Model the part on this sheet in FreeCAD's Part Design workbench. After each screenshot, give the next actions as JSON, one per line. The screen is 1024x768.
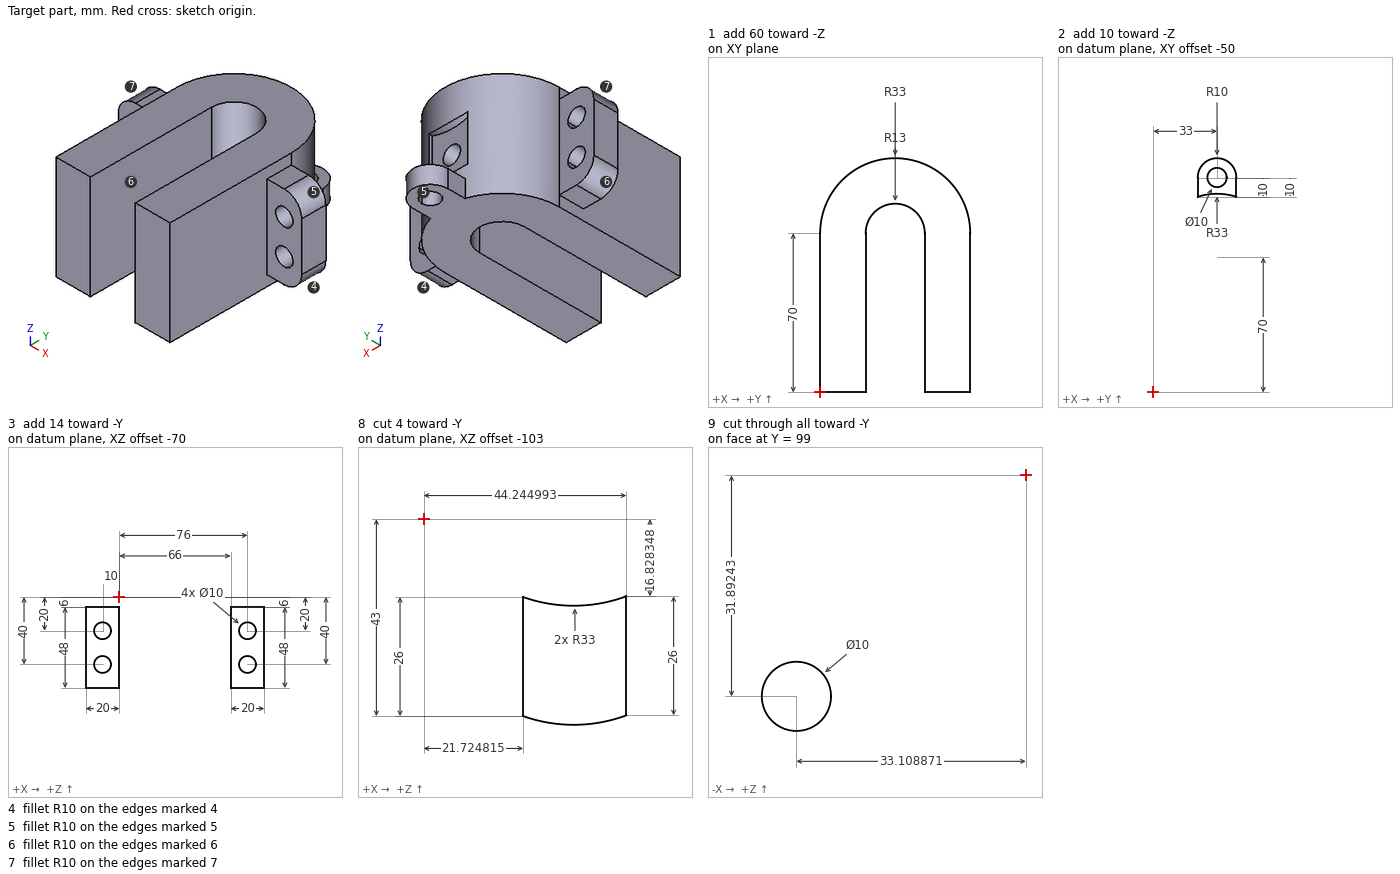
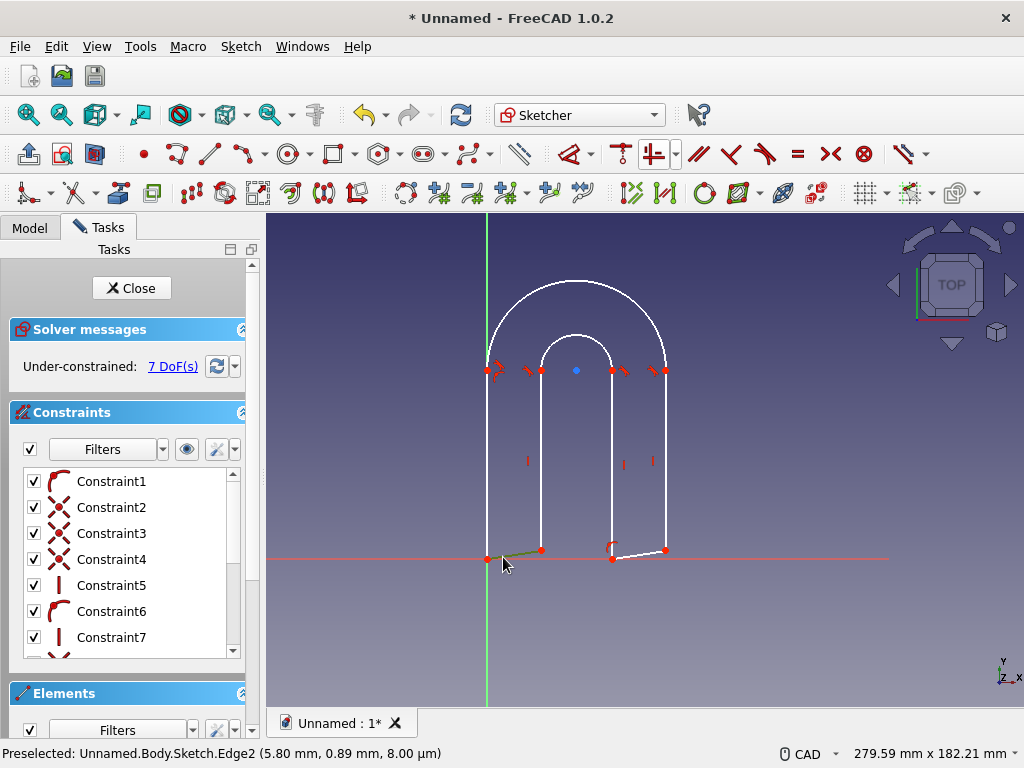
{"action": "key", "text": "h"}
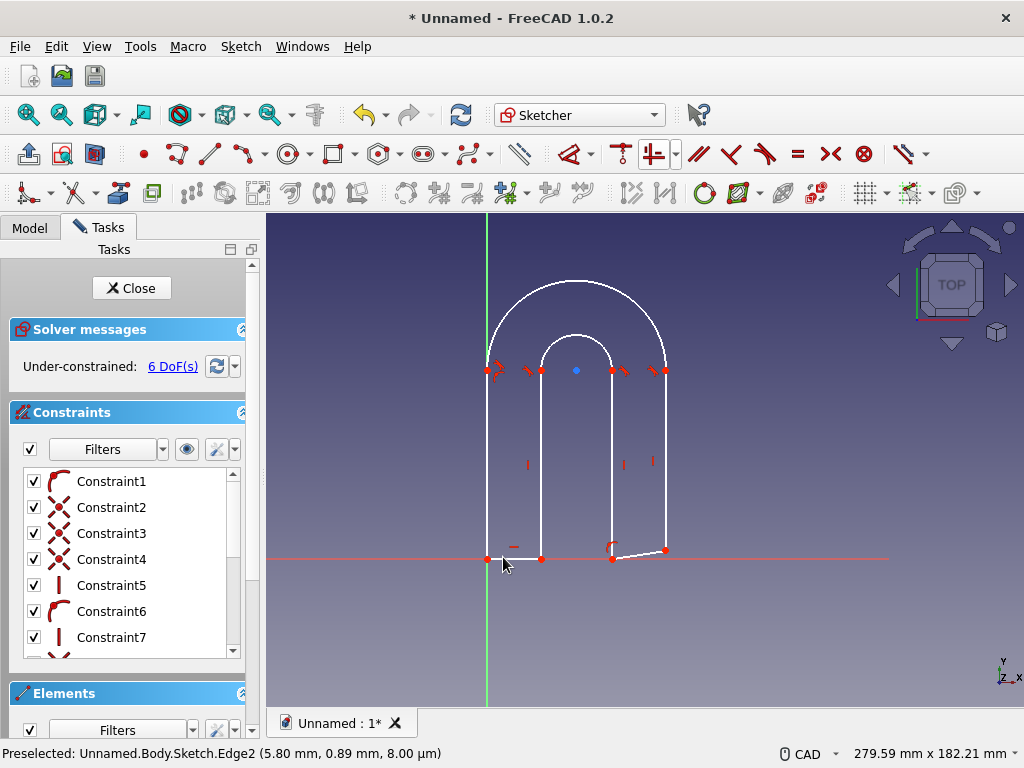
{"action": "left_click", "coordinate": [628, 557]}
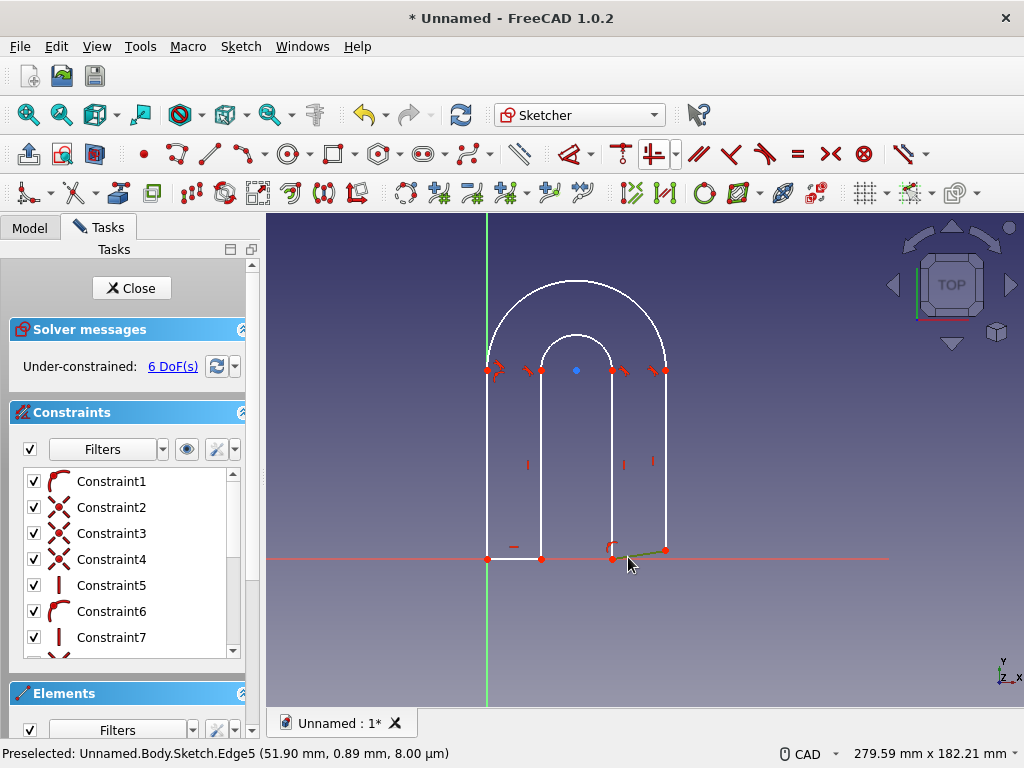
{"action": "key", "text": "h"}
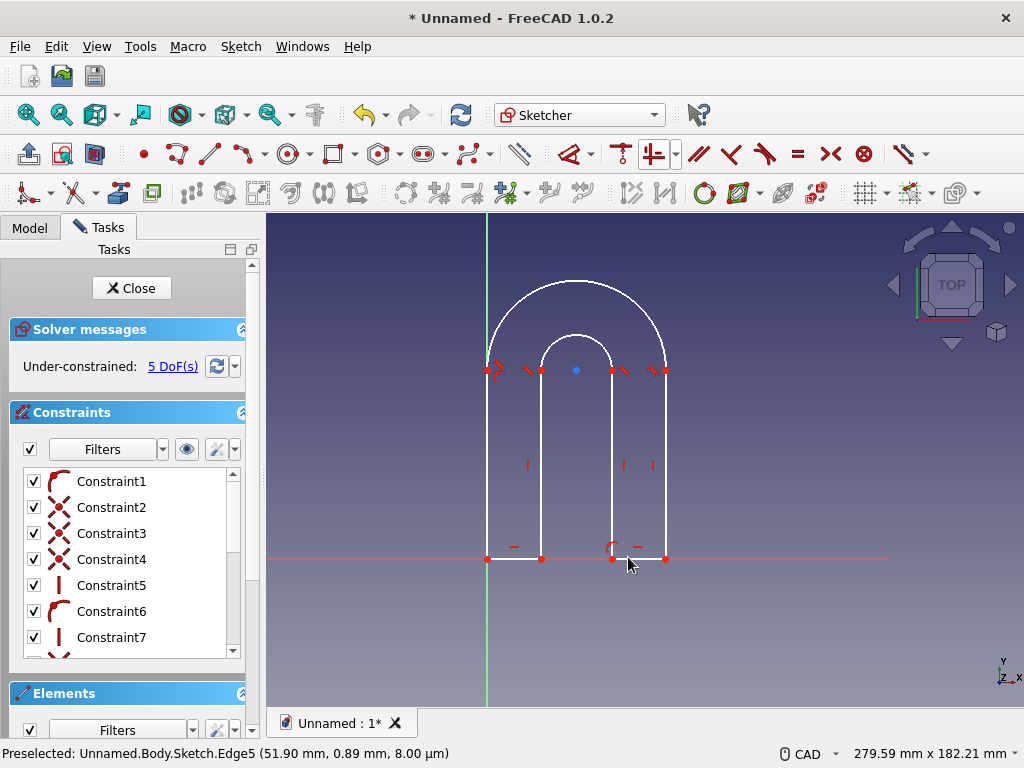
{"action": "left_click", "coordinate": [597, 342]}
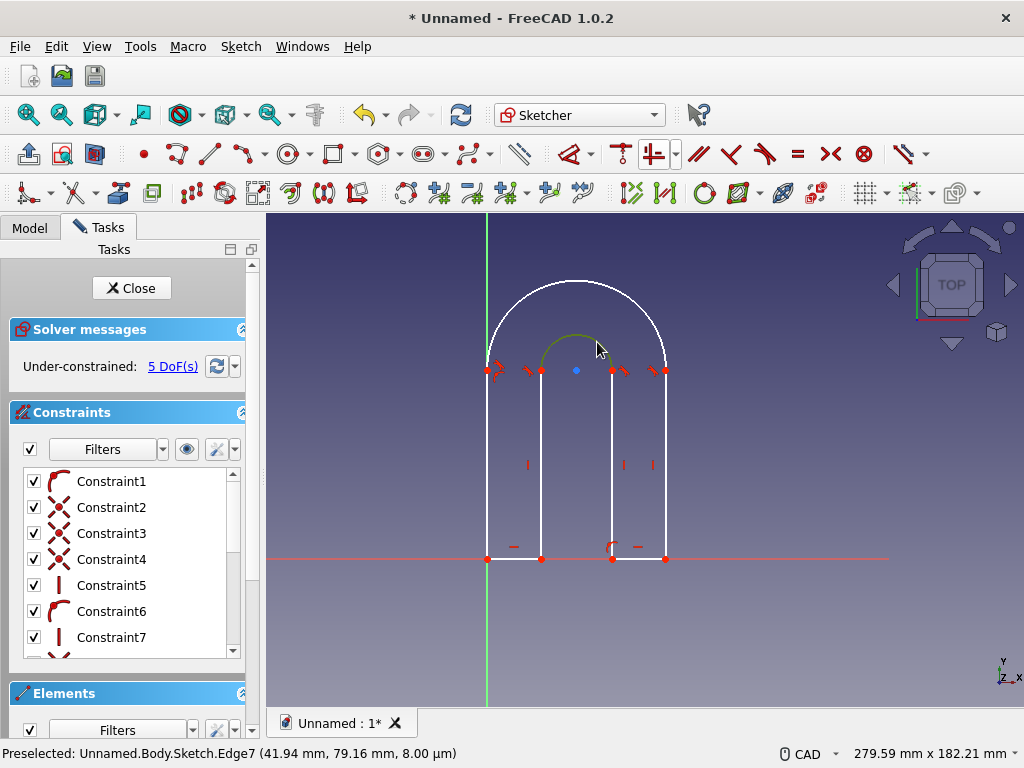
{"action": "left_click", "coordinate": [629, 298]}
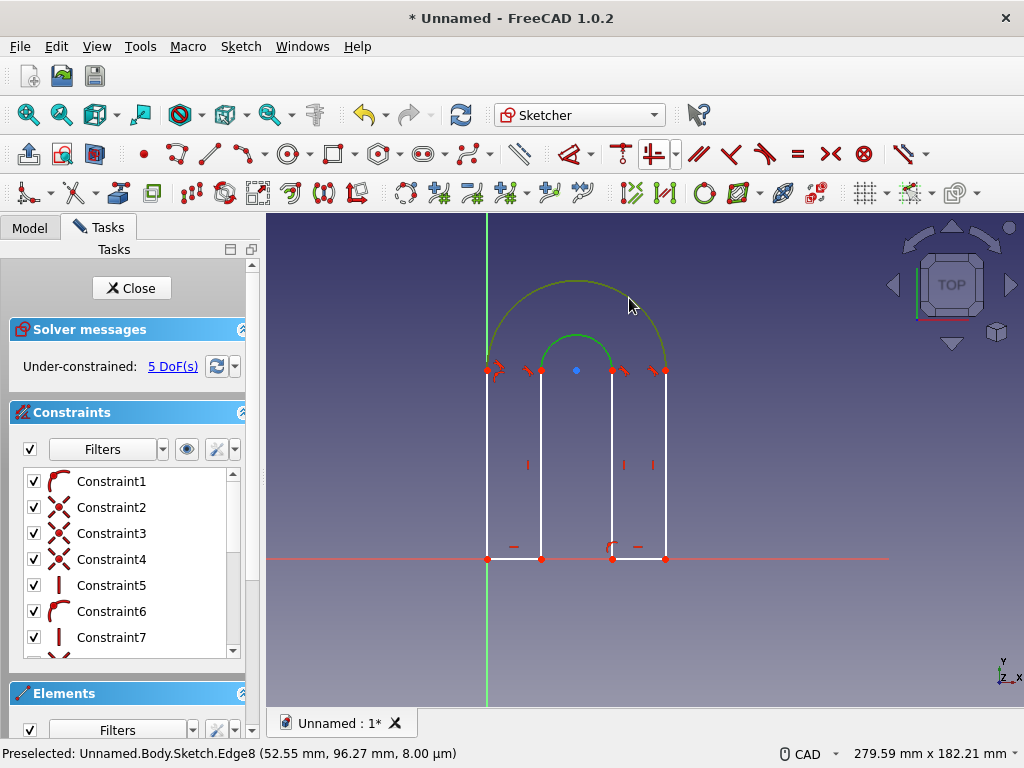
{"action": "left_click", "coordinate": [621, 154]}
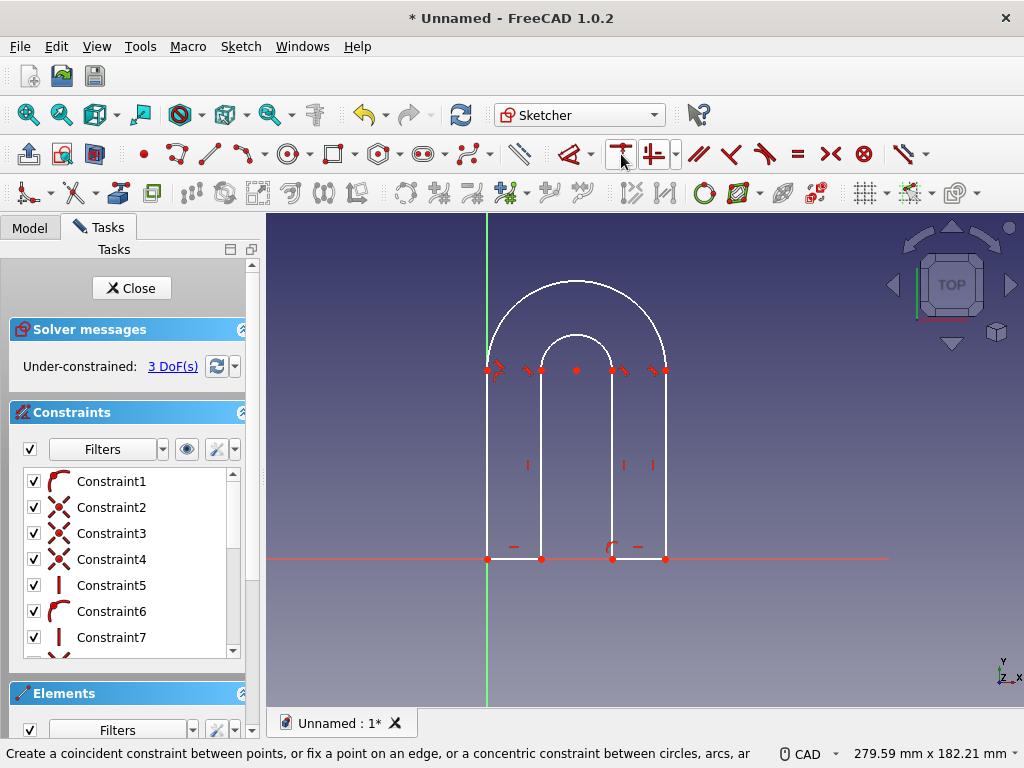
{"action": "left_click", "coordinate": [568, 154]}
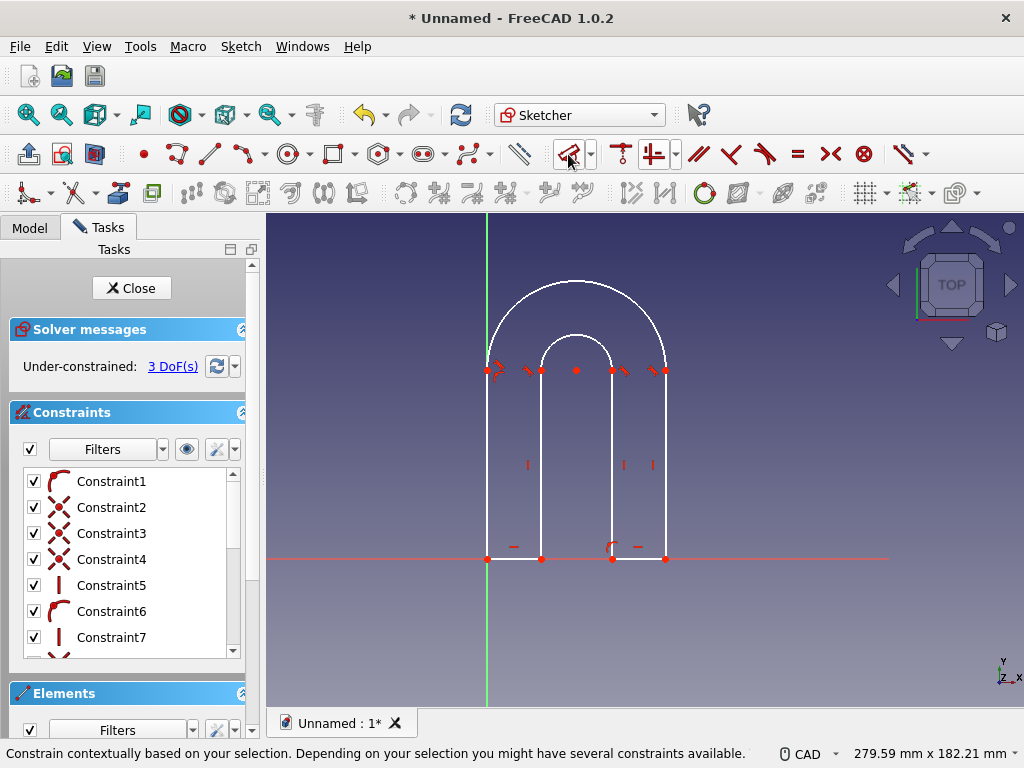
{"action": "left_click", "coordinate": [597, 342]}
{"action": "left_click", "coordinate": [616, 316]}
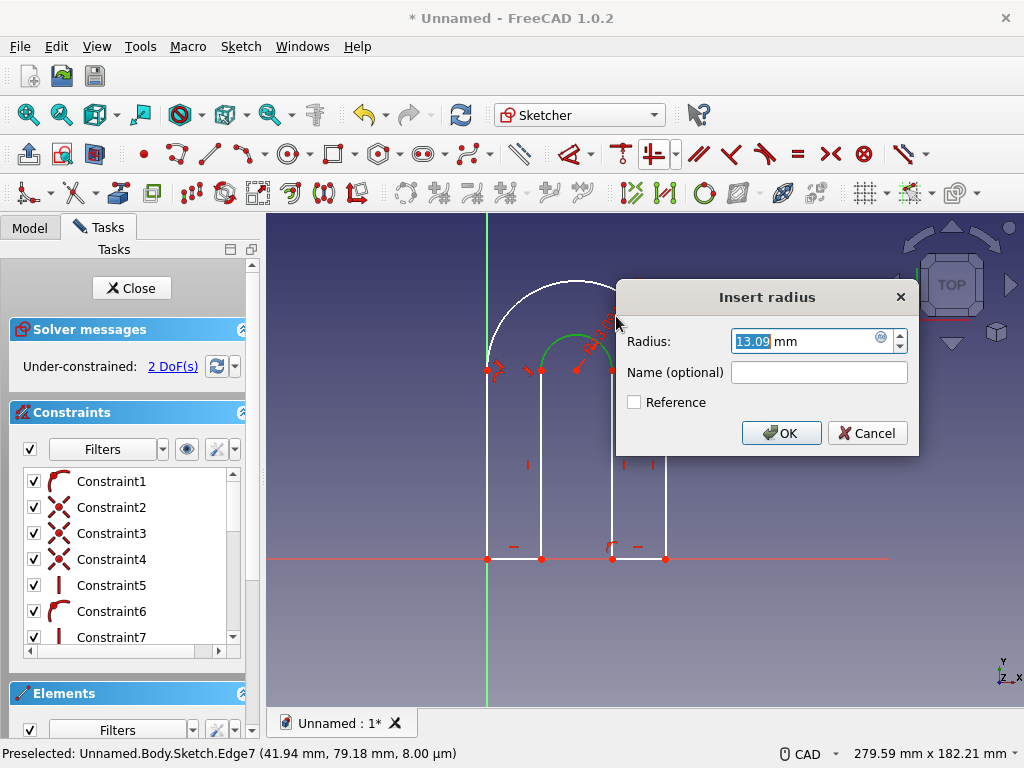
{"action": "type", "text": "13"}
{"action": "key", "text": "Return"}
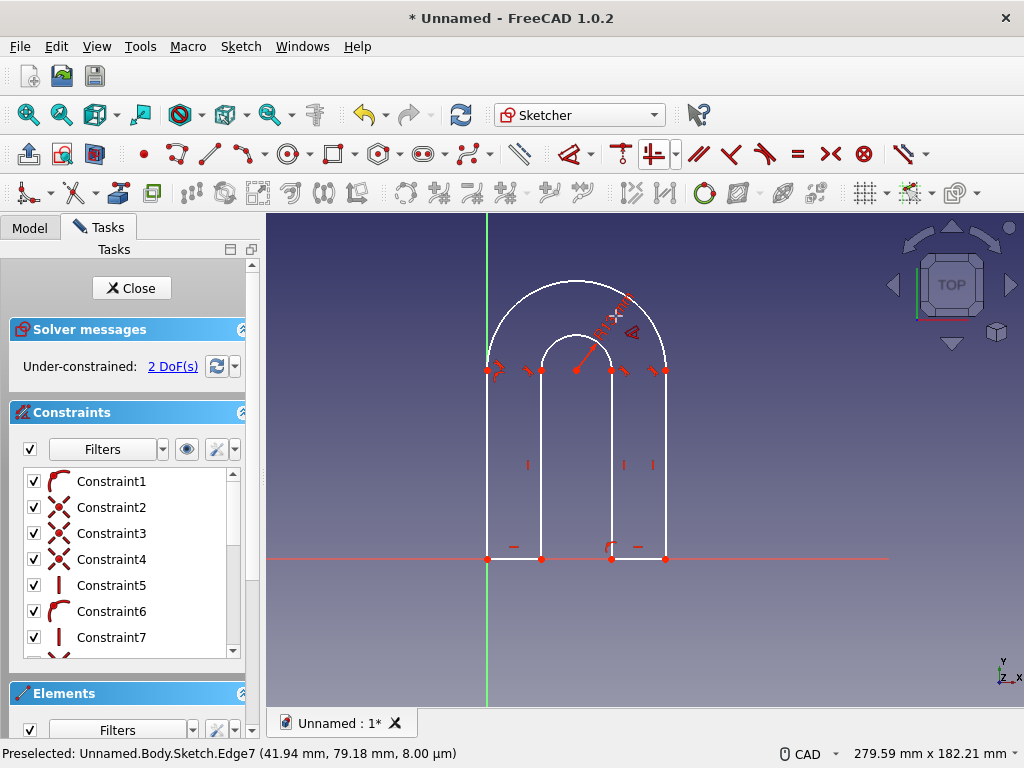
{"action": "left_click", "coordinate": [629, 298]}
{"action": "left_click", "coordinate": [648, 272]}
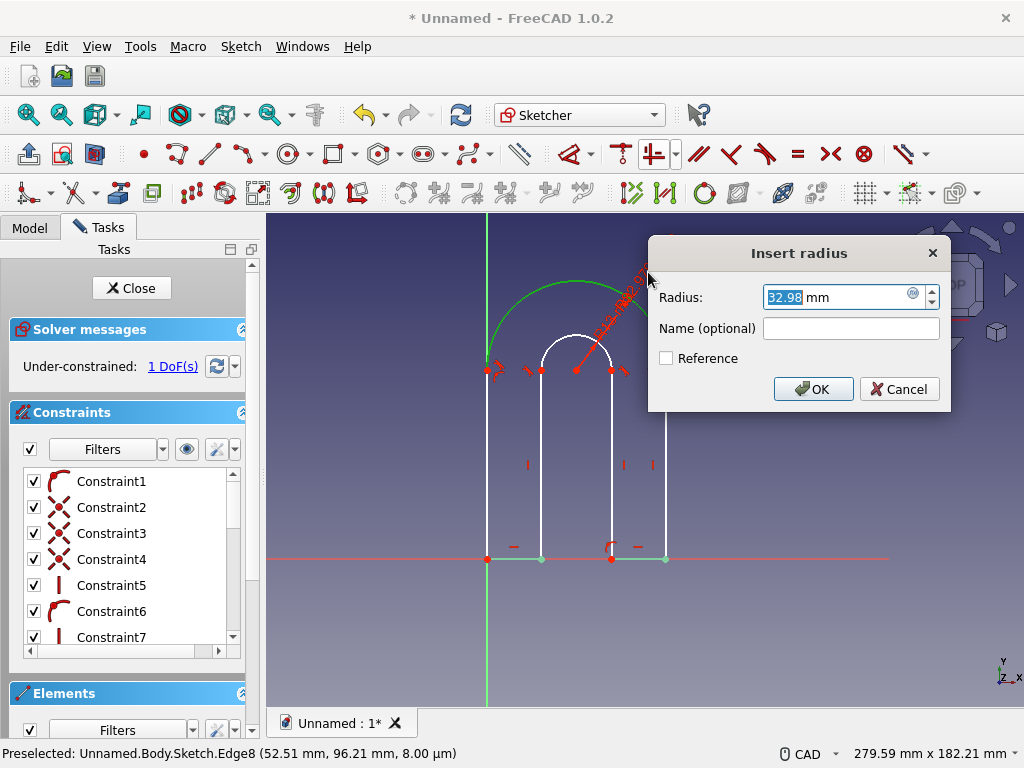
{"action": "type", "text": "33"}
{"action": "key", "text": "Return"}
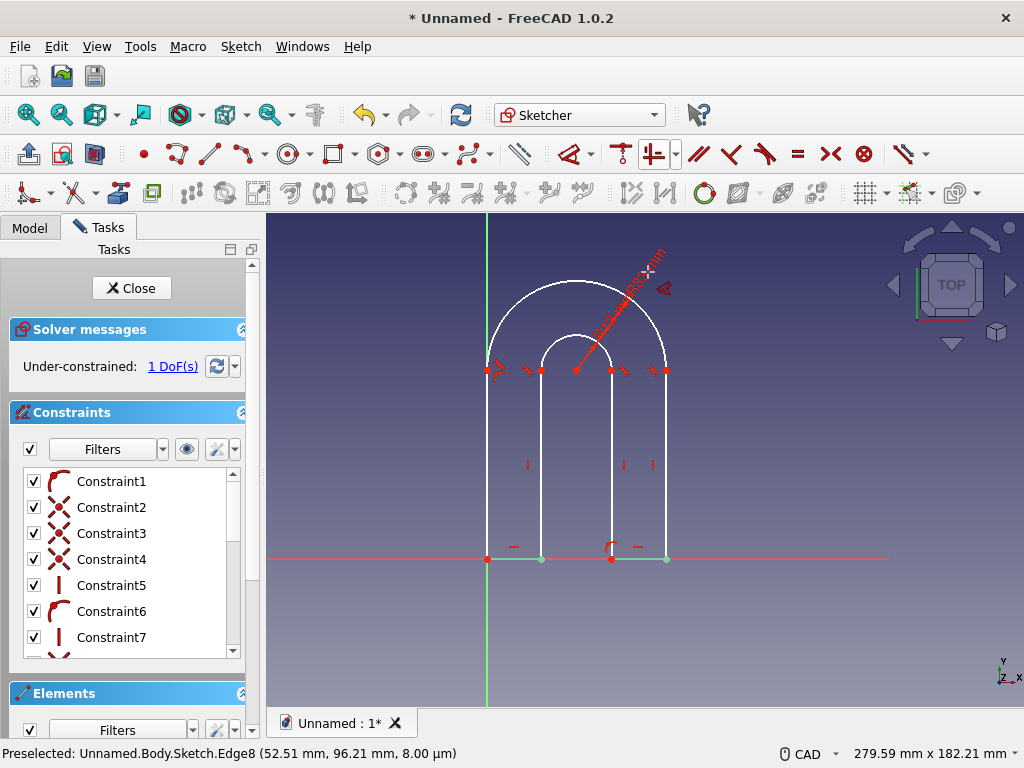
{"action": "left_click", "coordinate": [487, 427]}
{"action": "left_click", "coordinate": [453, 465]}